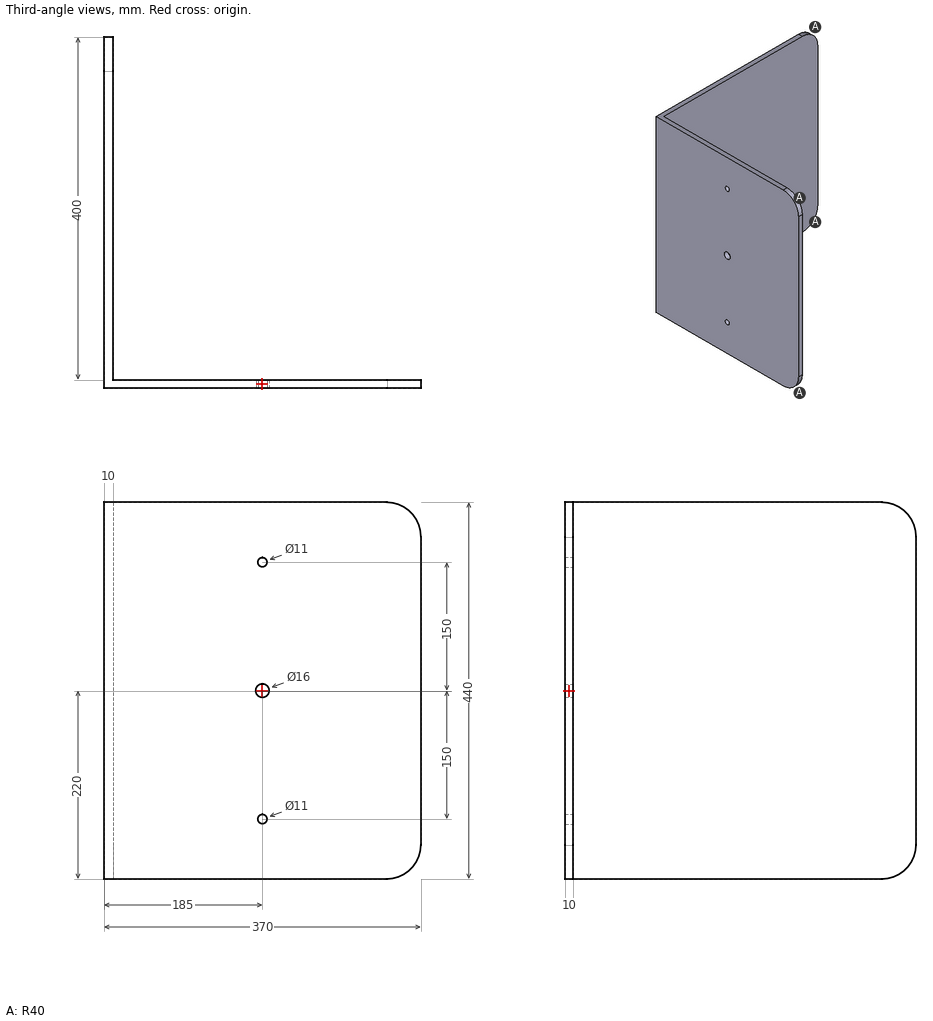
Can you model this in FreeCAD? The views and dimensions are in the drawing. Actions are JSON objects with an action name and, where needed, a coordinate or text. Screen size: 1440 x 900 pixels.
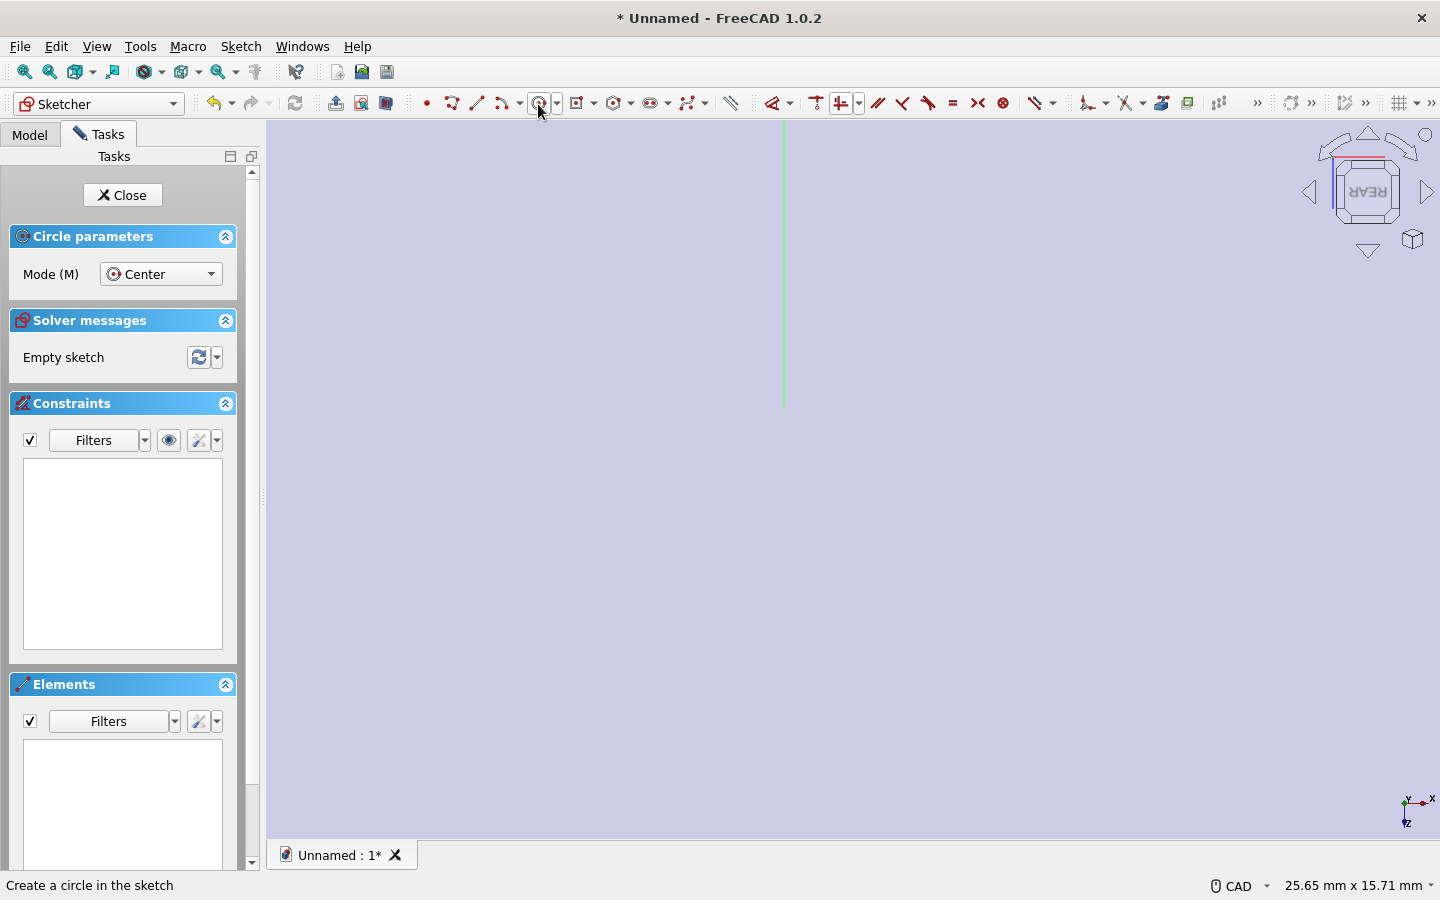
{"action": "left_click", "coordinate": [784, 480]}
{"action": "mouse_move", "coordinate": [962, 302]}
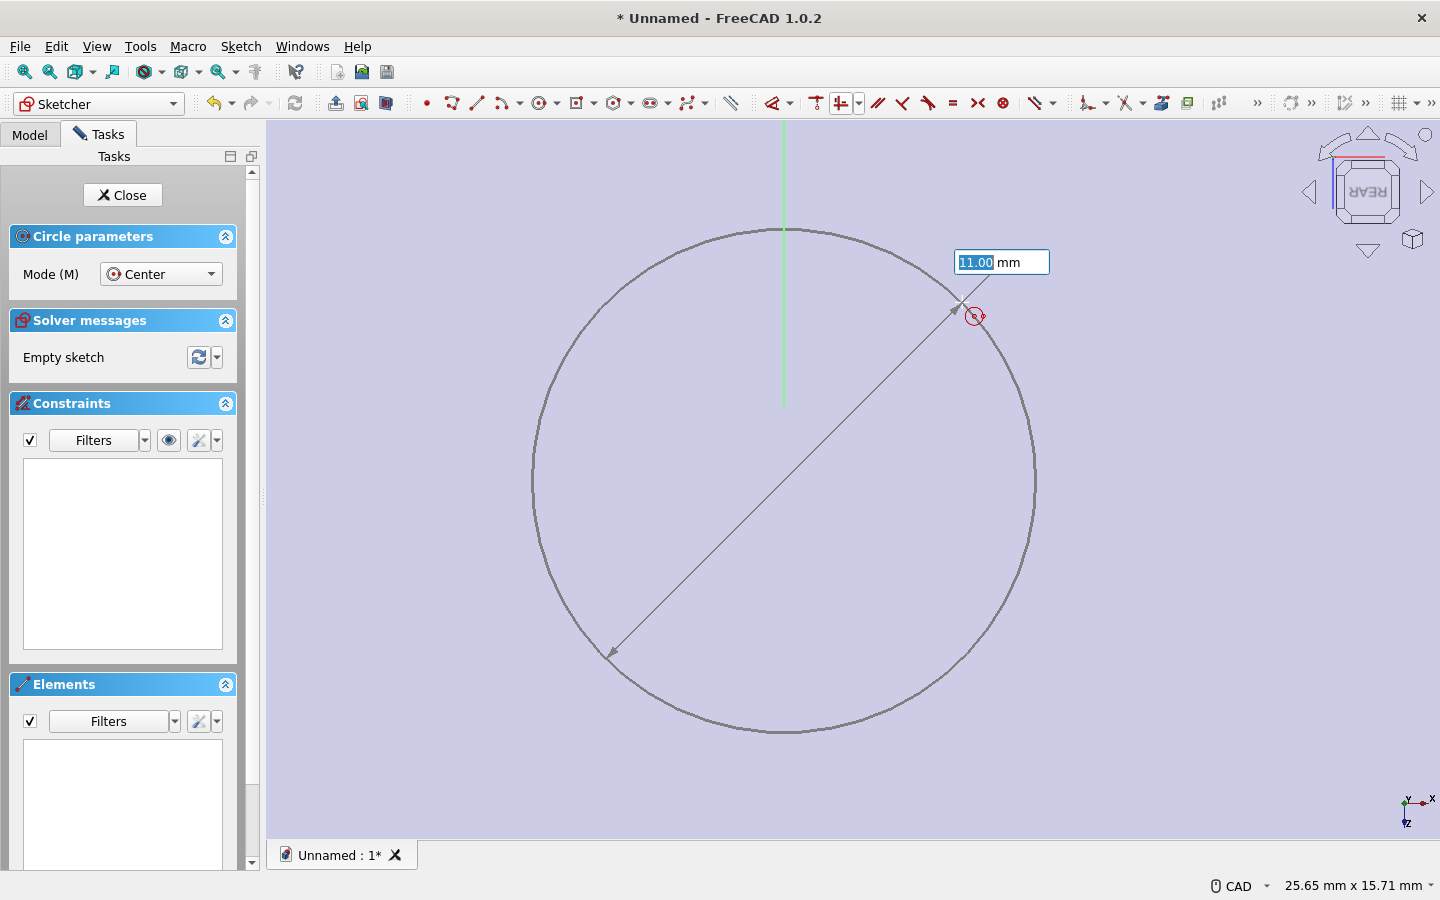
{"action": "type", "text": "11"}
{"action": "key", "text": "Return"}
{"action": "key", "text": "Escape"}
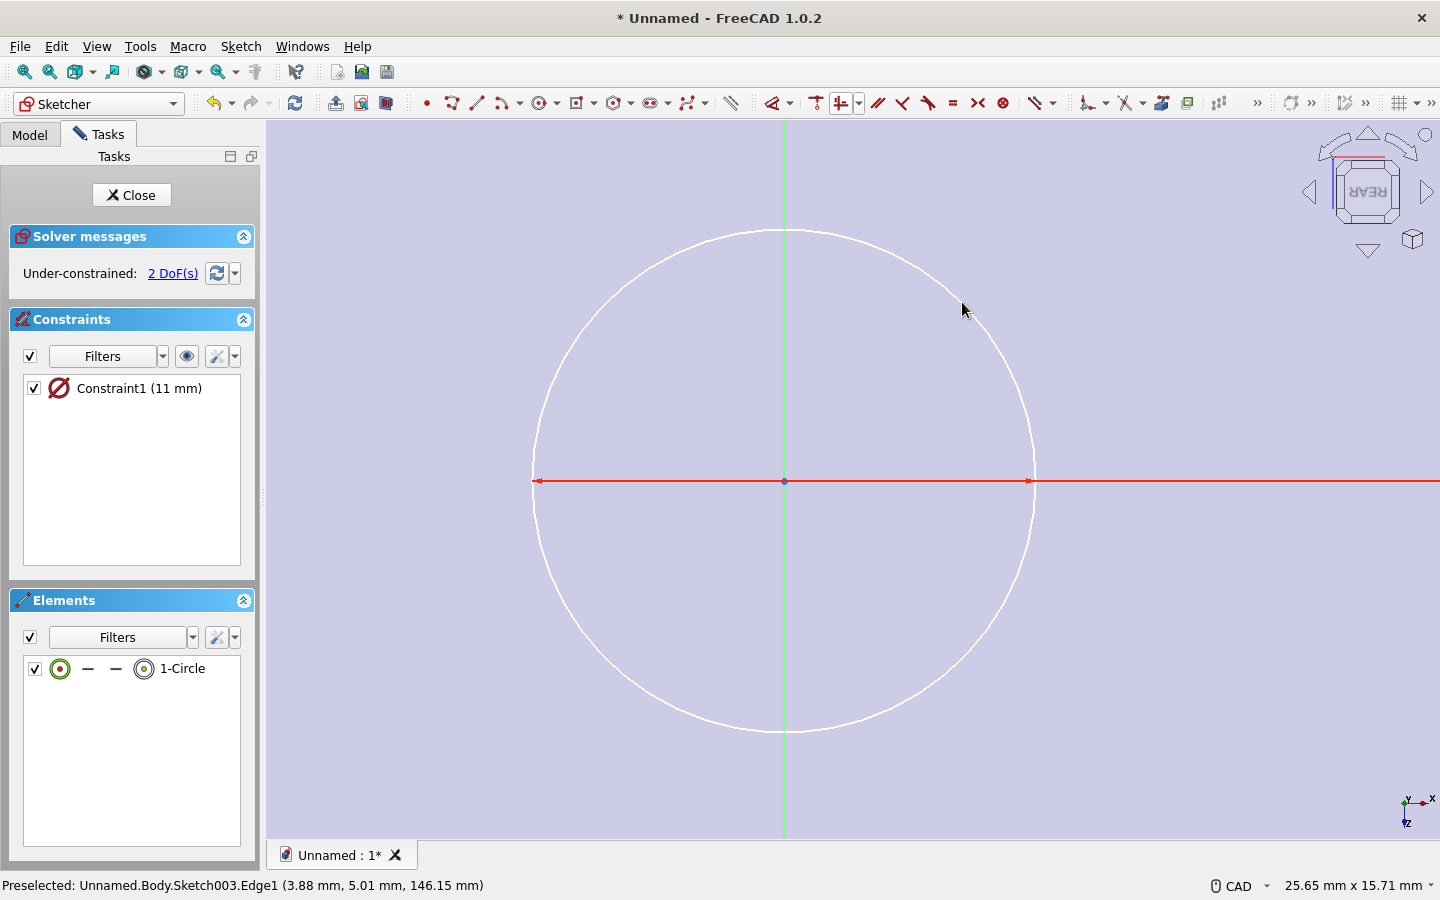
{"action": "left_click", "coordinate": [784, 481]}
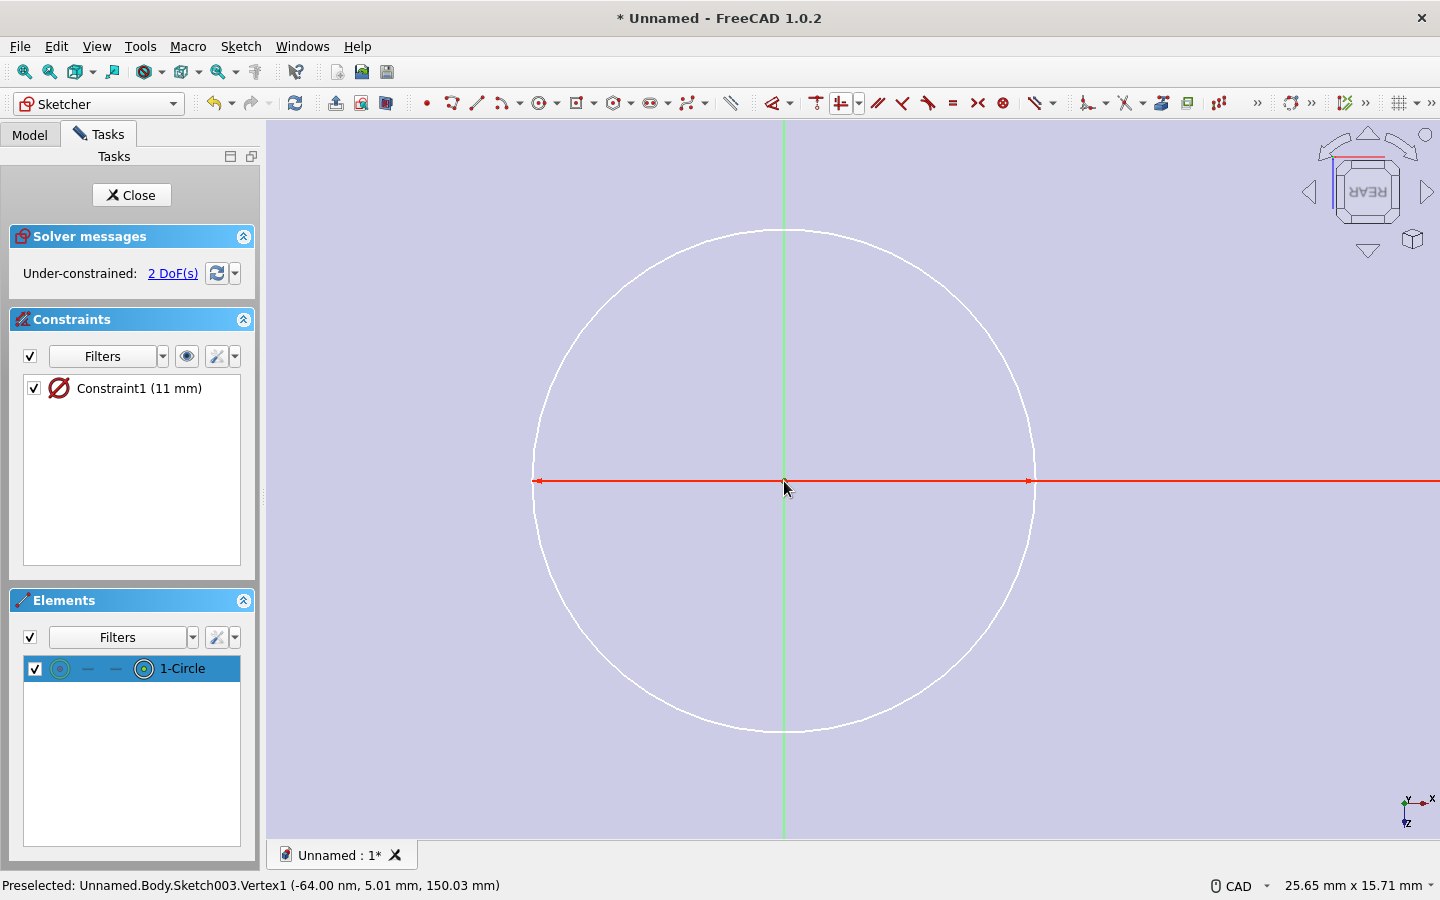
{"action": "left_click", "coordinate": [784, 764]}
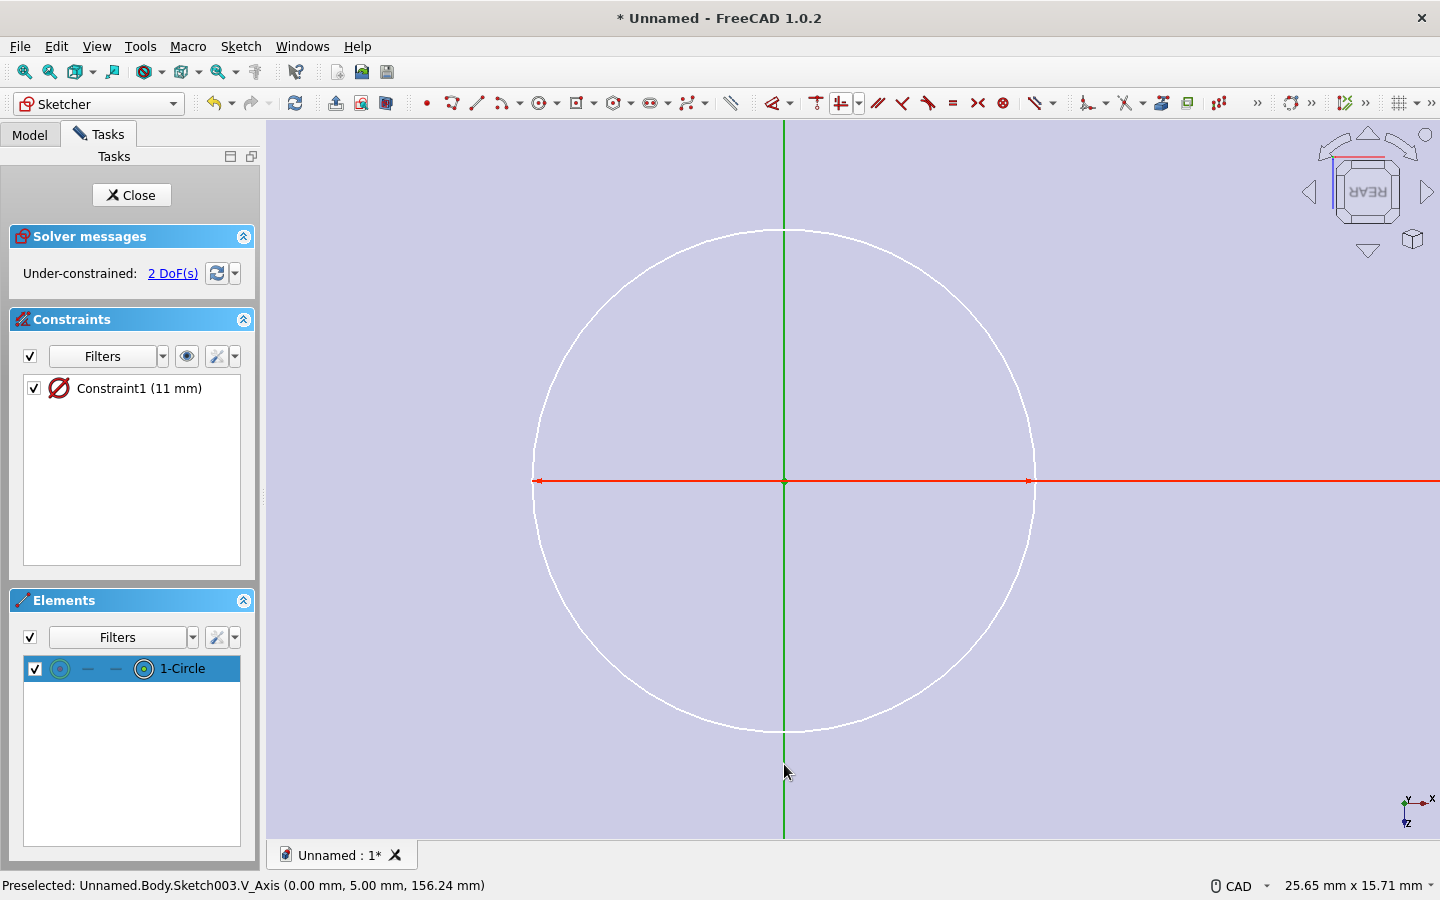
{"action": "left_click", "coordinate": [816, 104]}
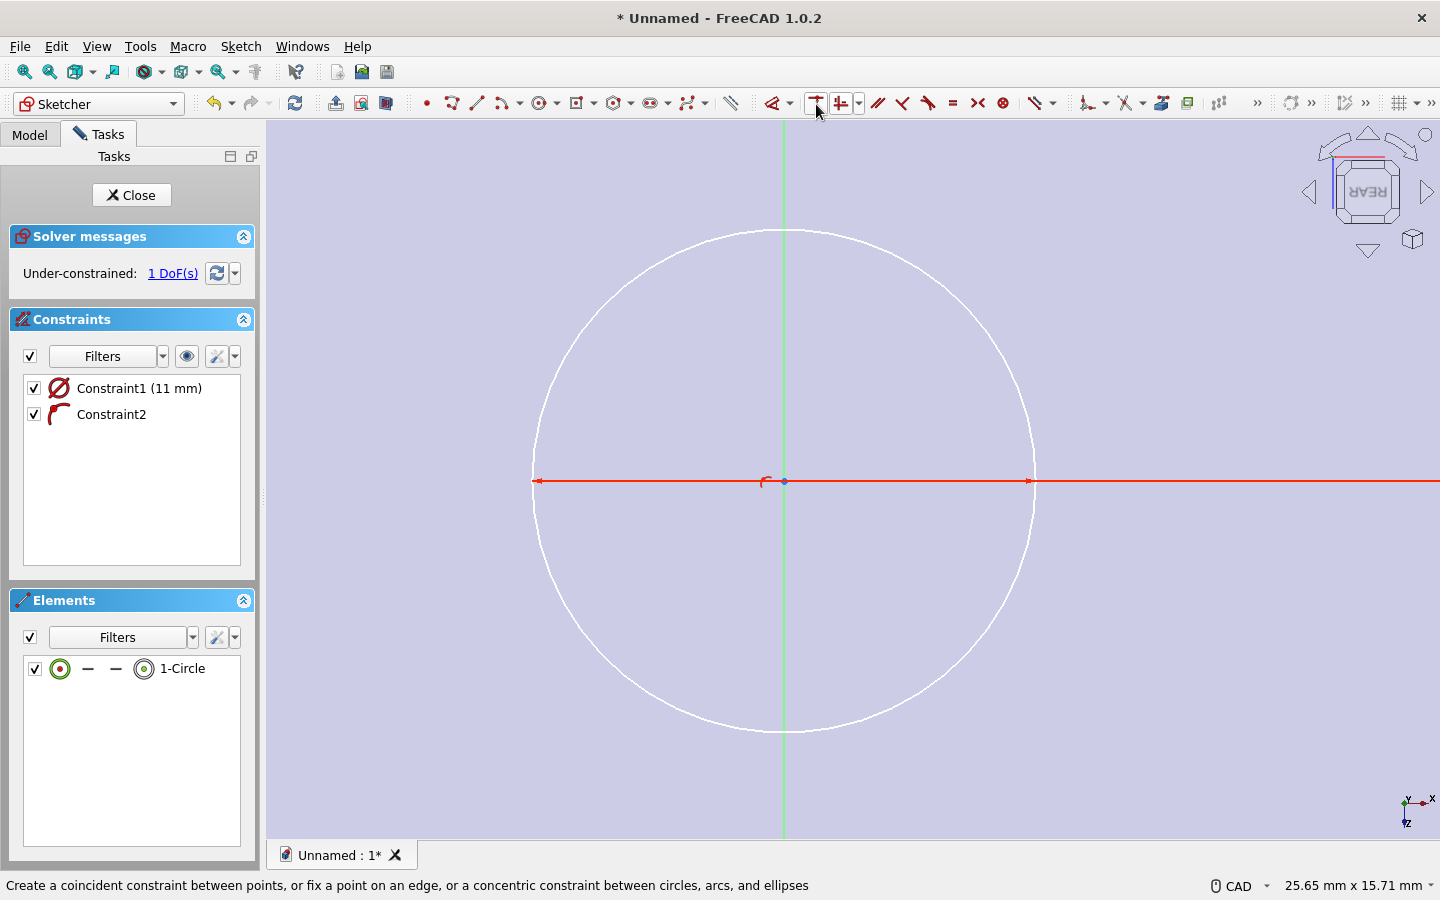
{"action": "left_click", "coordinate": [772, 104]}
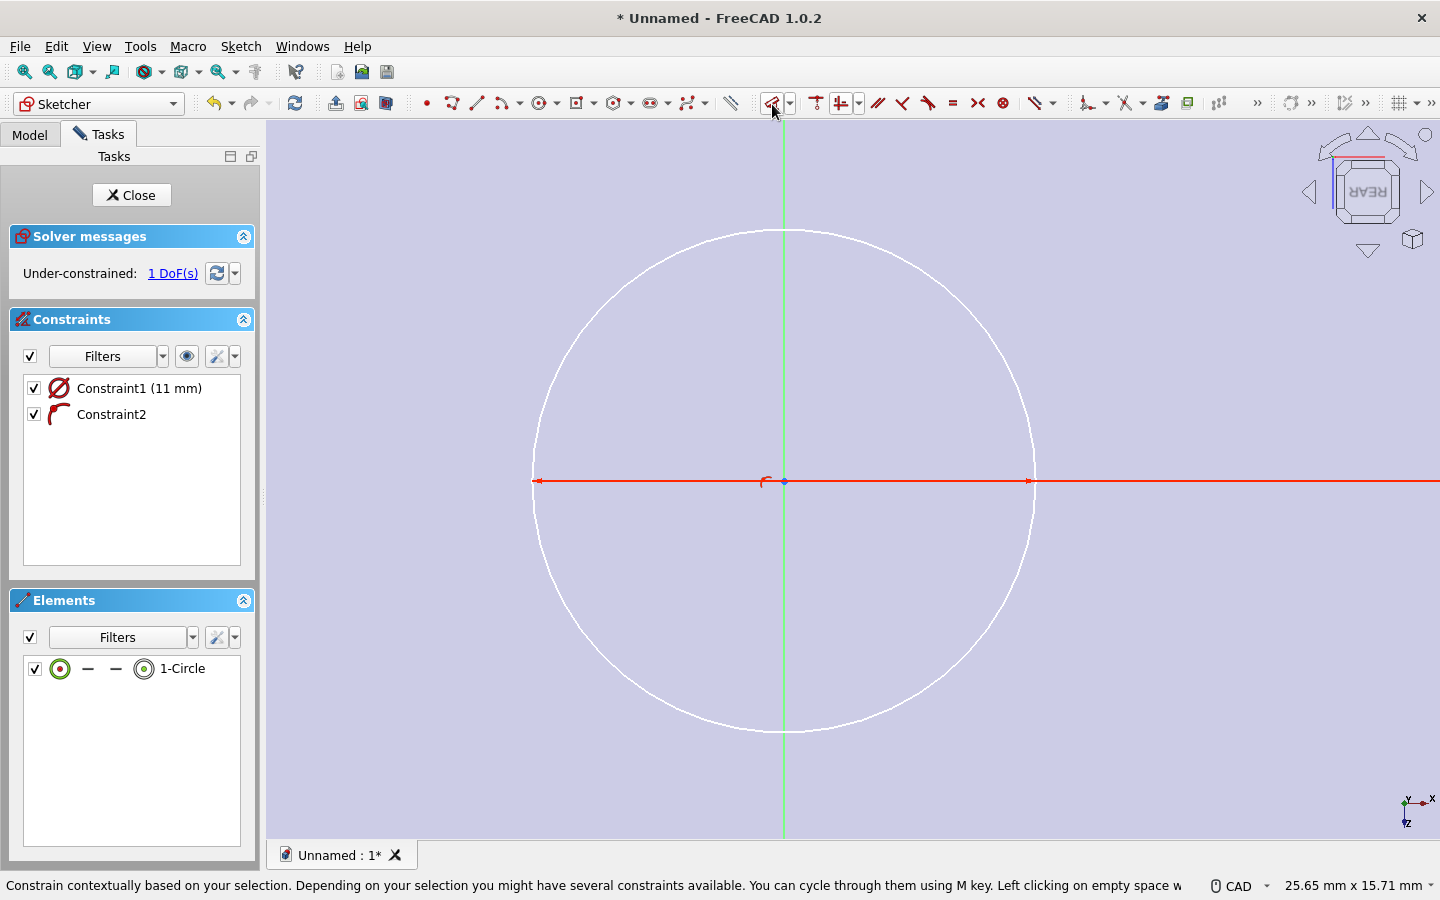
{"action": "left_click", "coordinate": [784, 481]}
{"action": "left_click", "coordinate": [818, 314]}